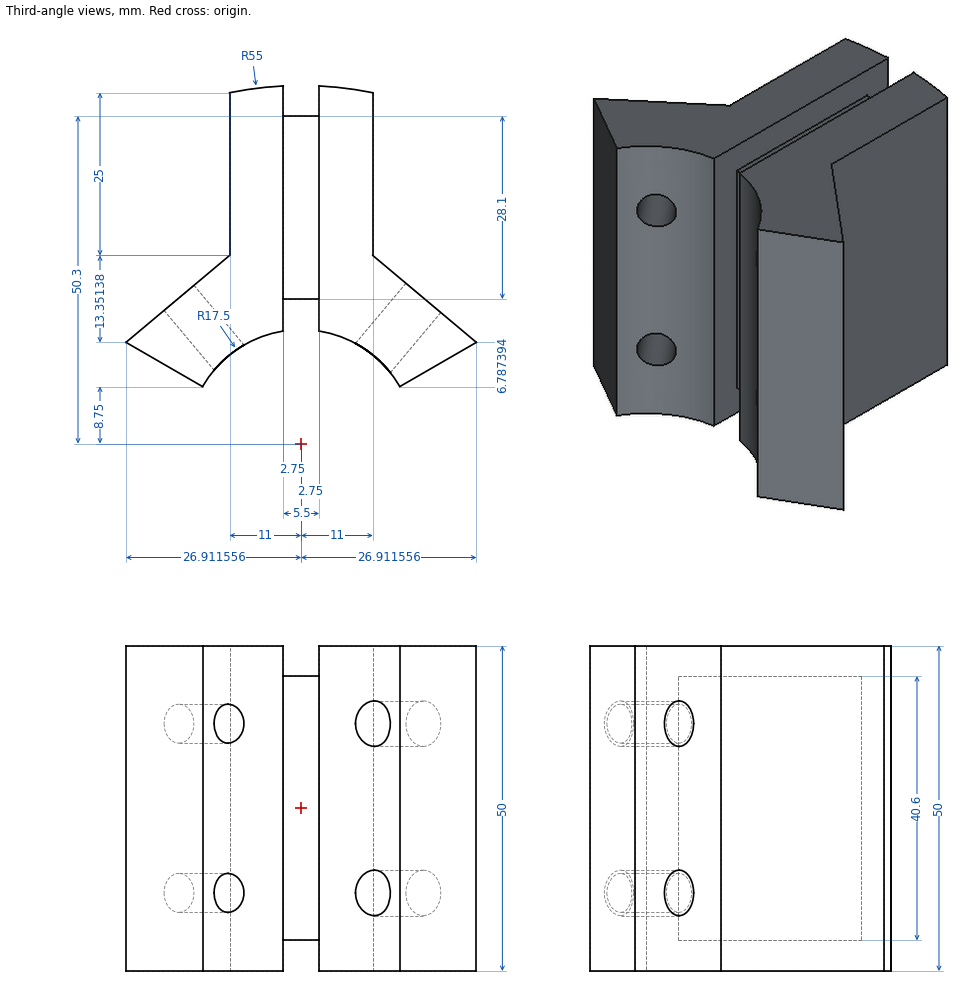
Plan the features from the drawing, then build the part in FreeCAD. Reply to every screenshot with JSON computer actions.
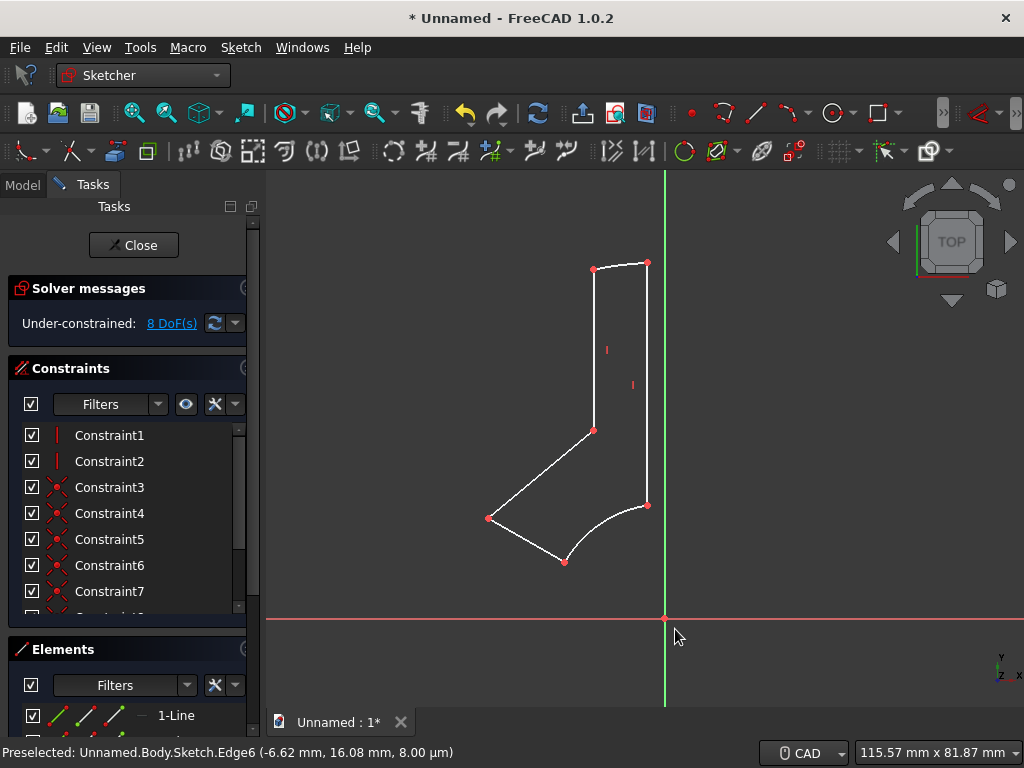
{"action": "left_click", "coordinate": [631, 264]}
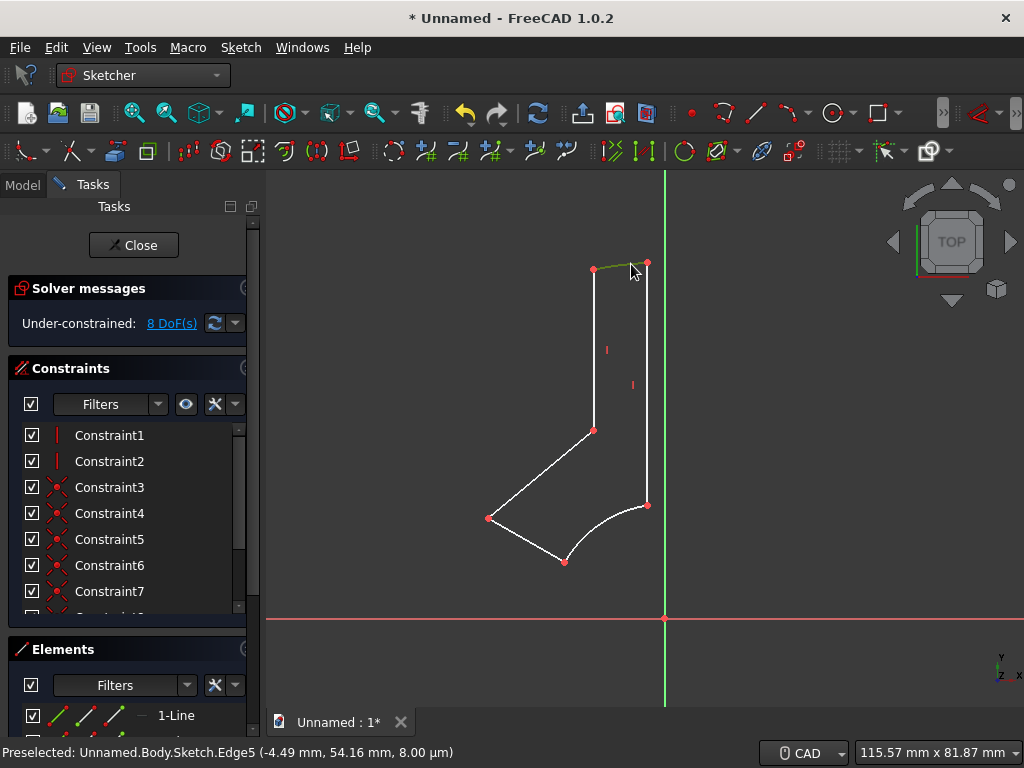
{"action": "left_click", "coordinate": [1002, 114]}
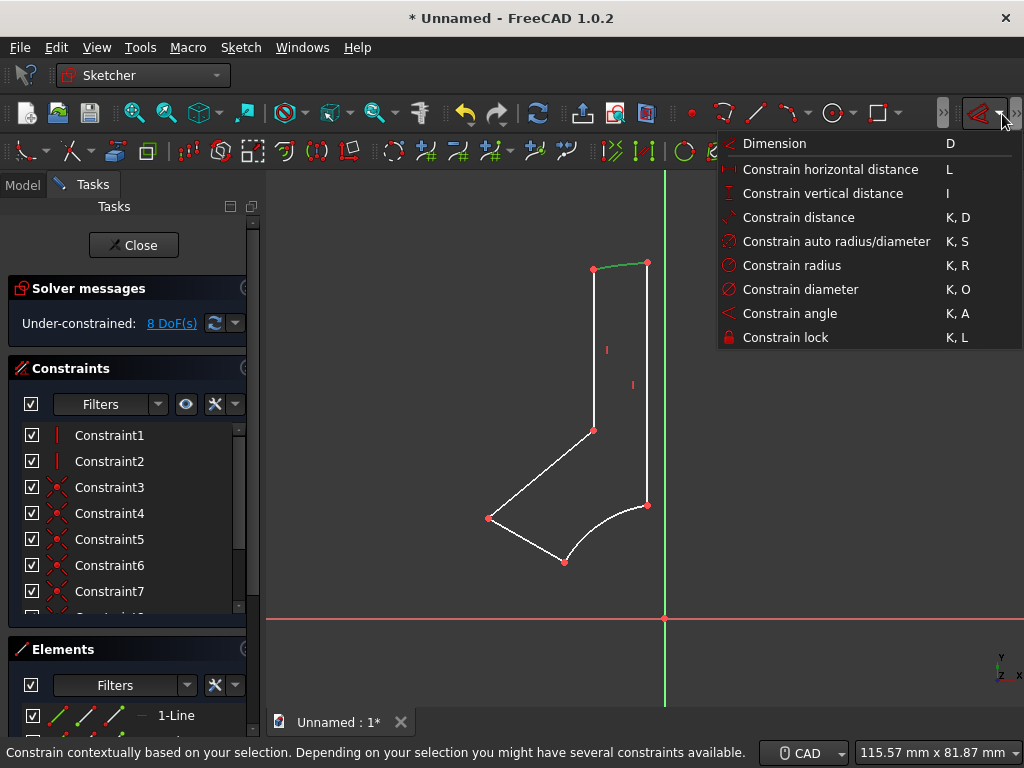
{"action": "left_click", "coordinate": [870, 265]}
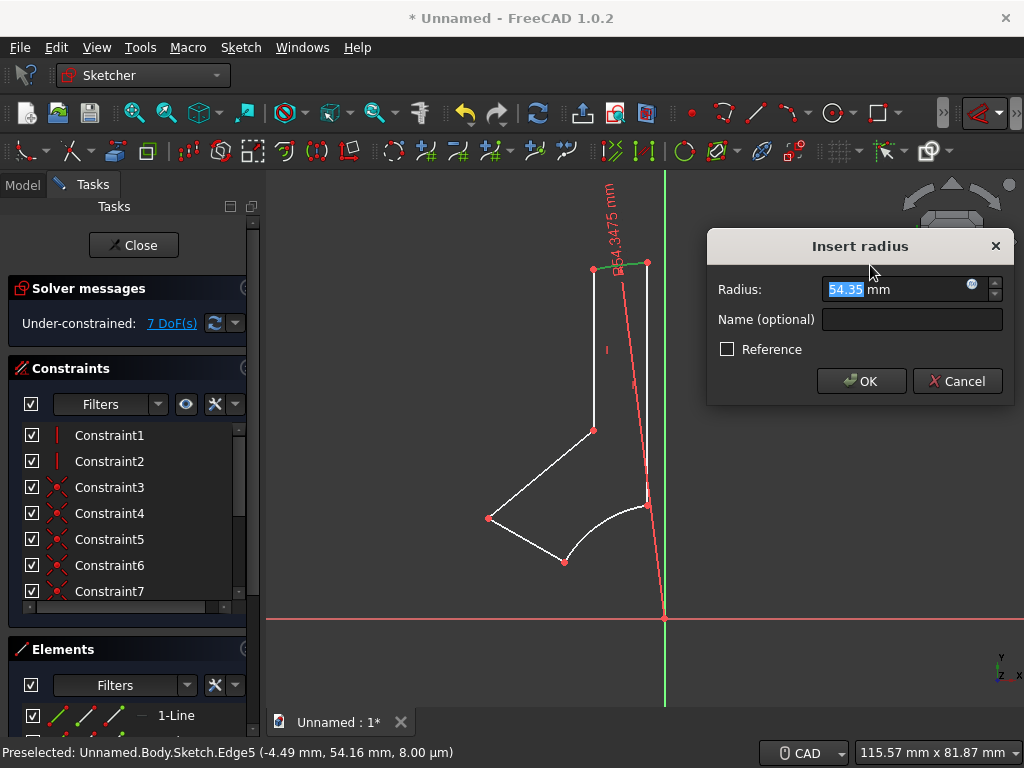
{"action": "type", "text": "55"}
{"action": "key", "text": "Return"}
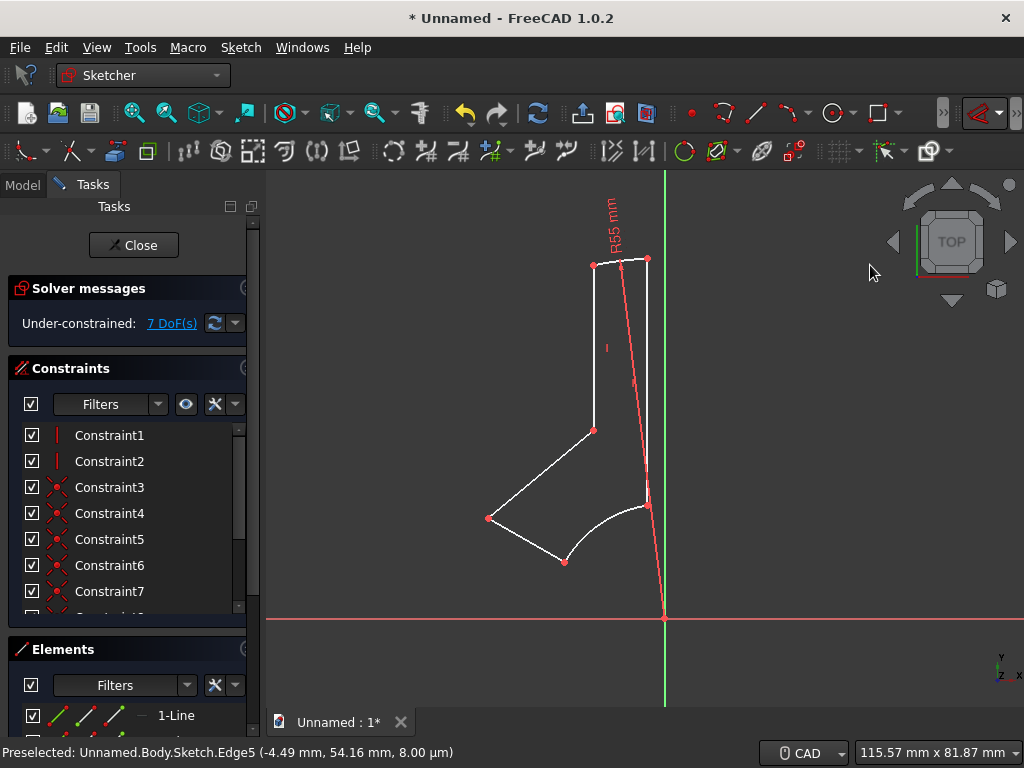
{"action": "left_click", "coordinate": [618, 514]}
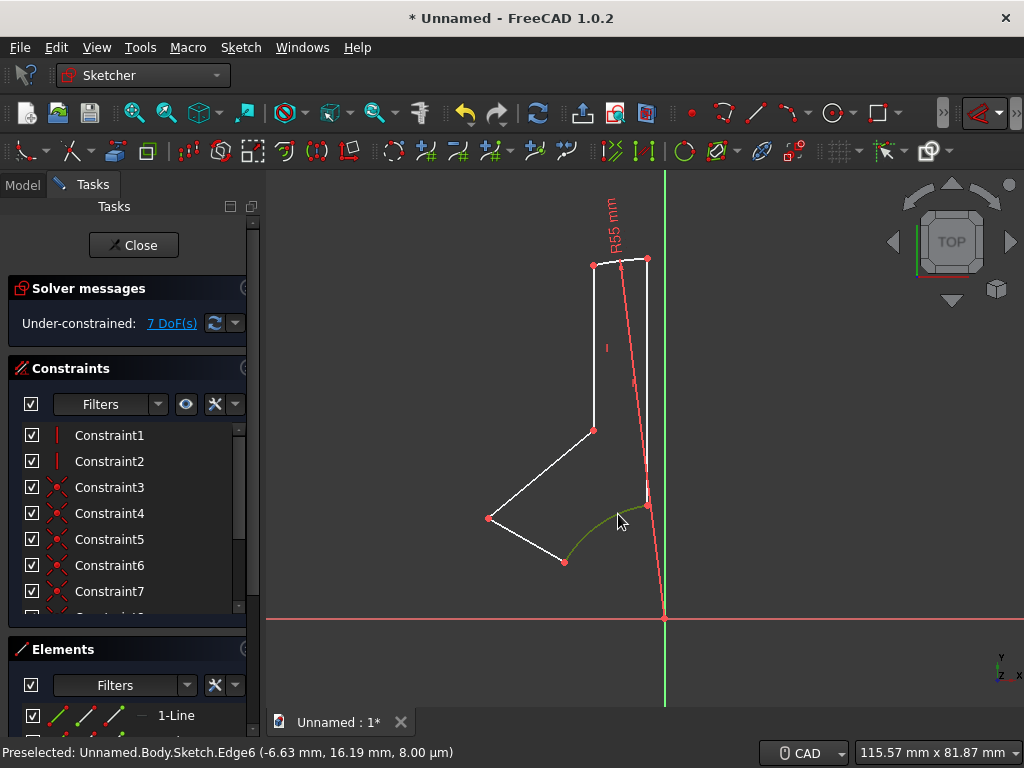
{"action": "key", "text": "k r"}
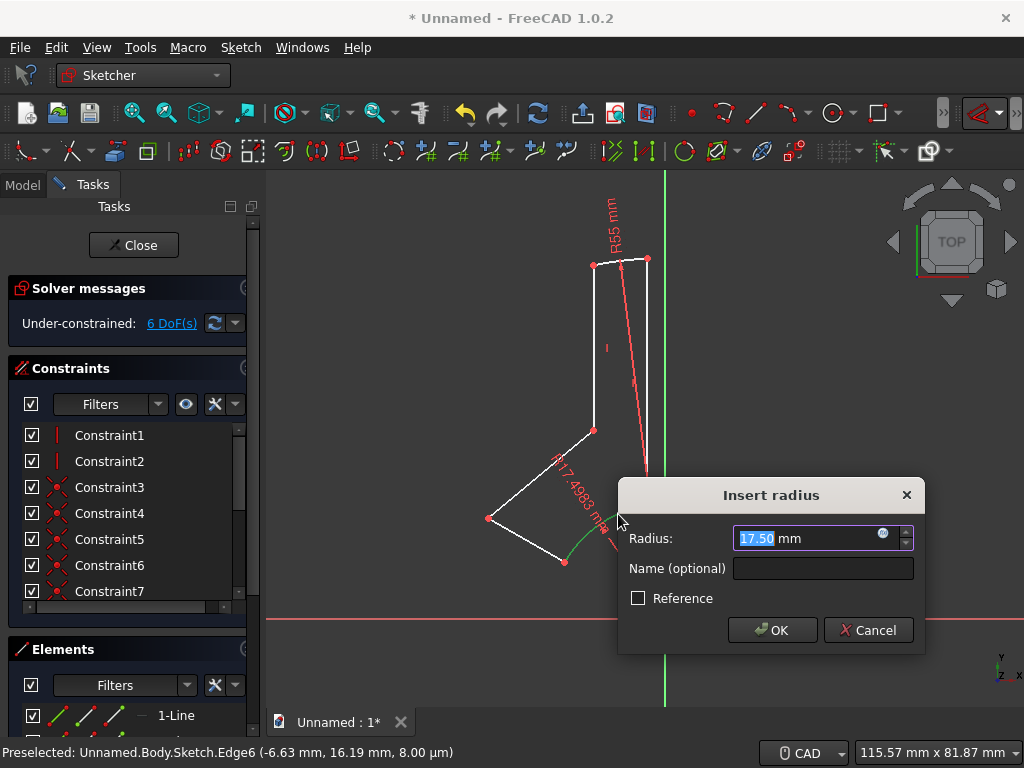
{"action": "type", "text": "17.5"}
{"action": "key", "text": "Return"}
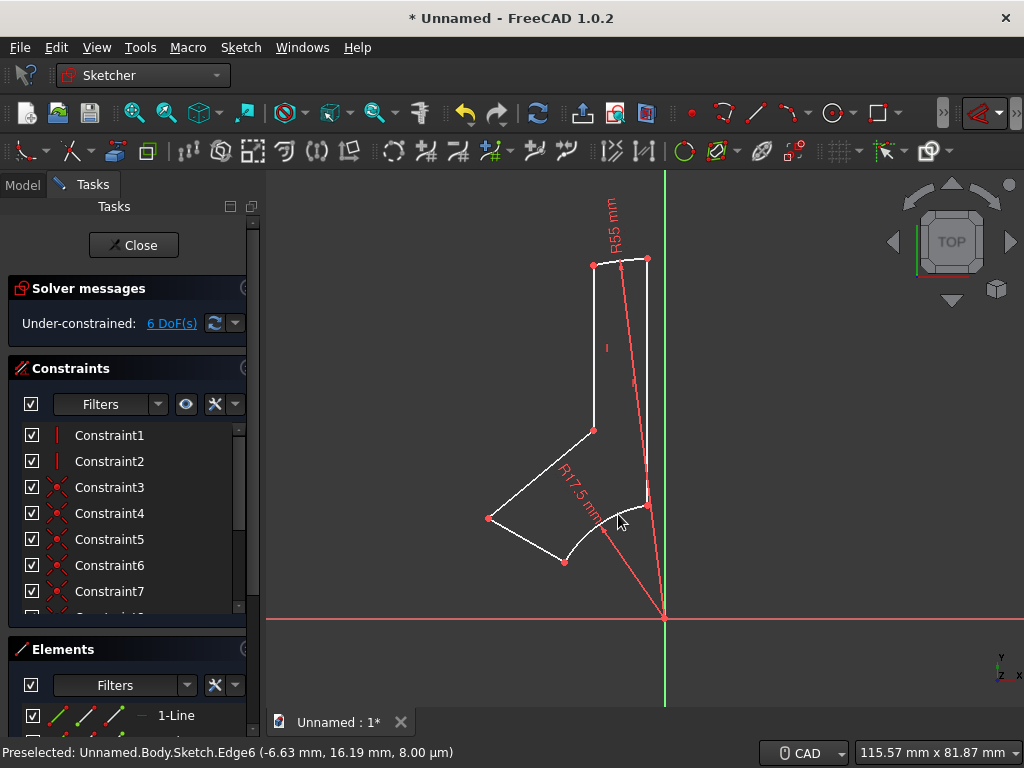
{"action": "left_click", "coordinate": [594, 315]}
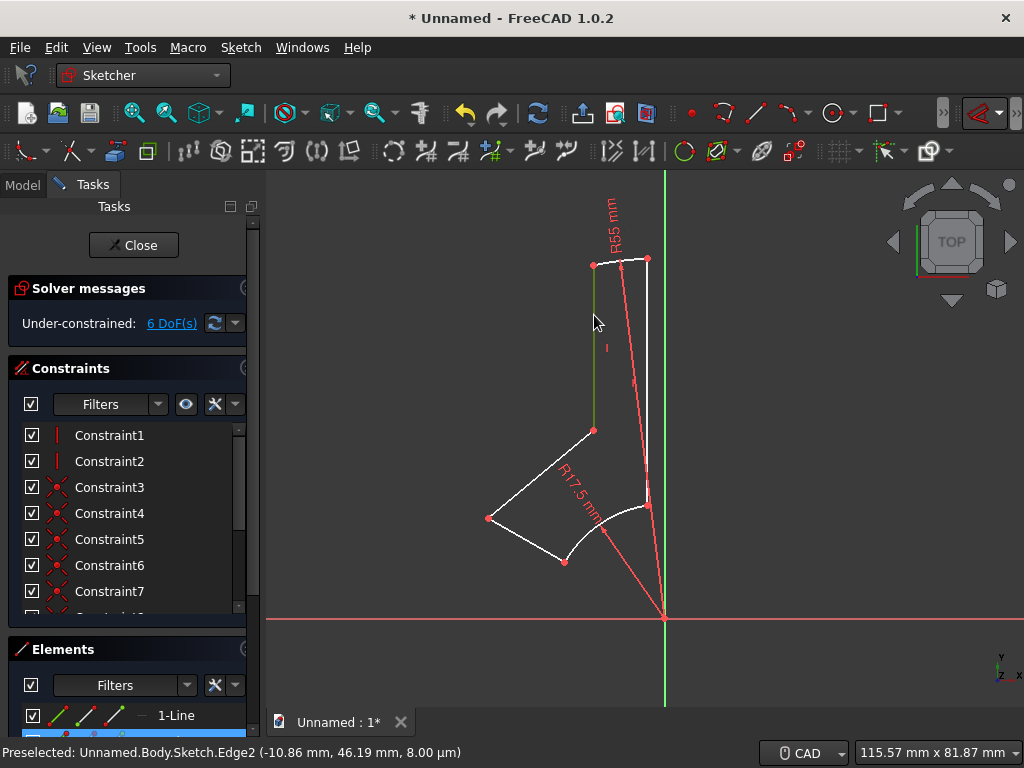
{"action": "left_click", "coordinate": [1002, 114]}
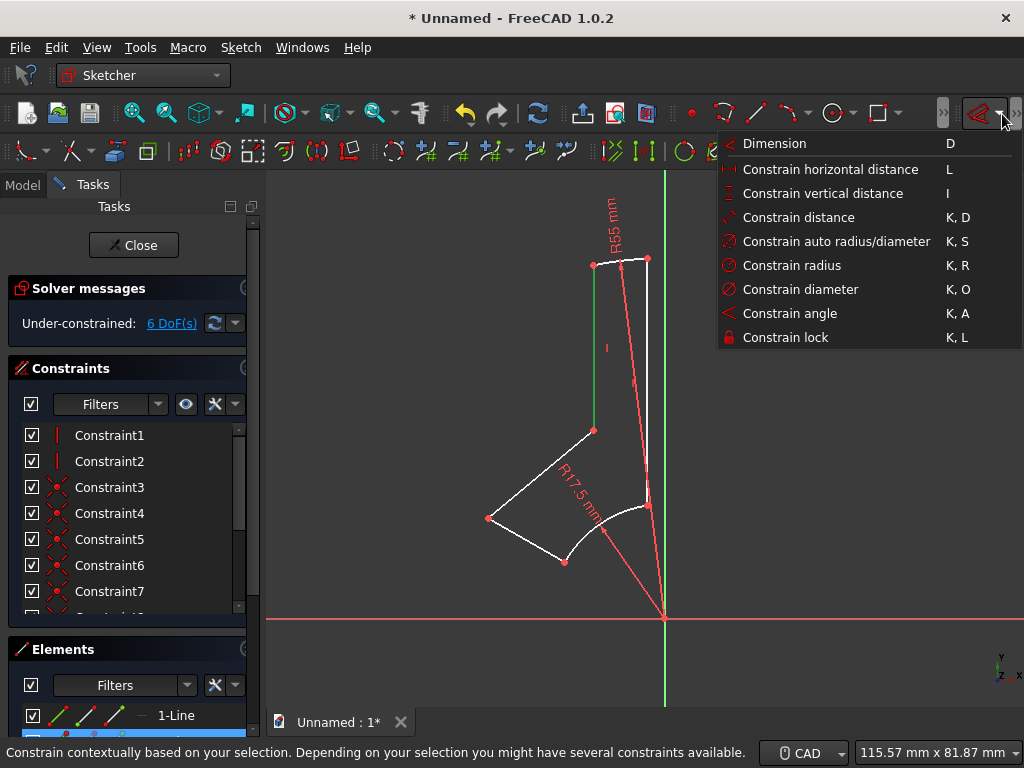
{"action": "left_click", "coordinate": [870, 193]}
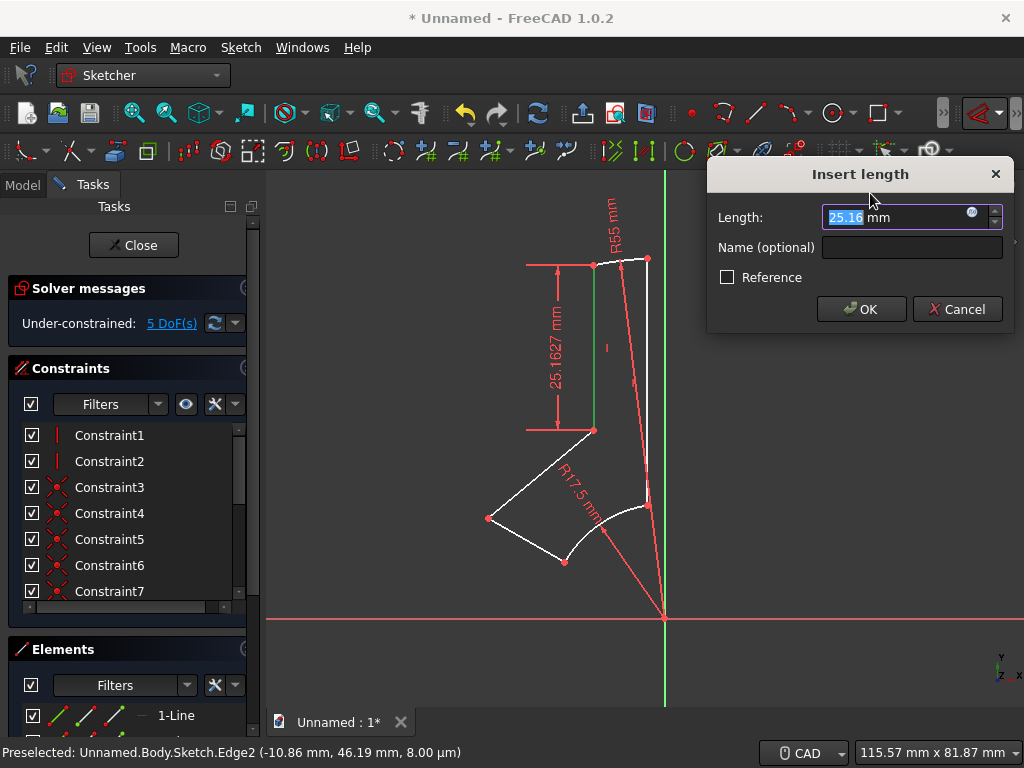
{"action": "type", "text": "25"}
{"action": "key", "text": "Return"}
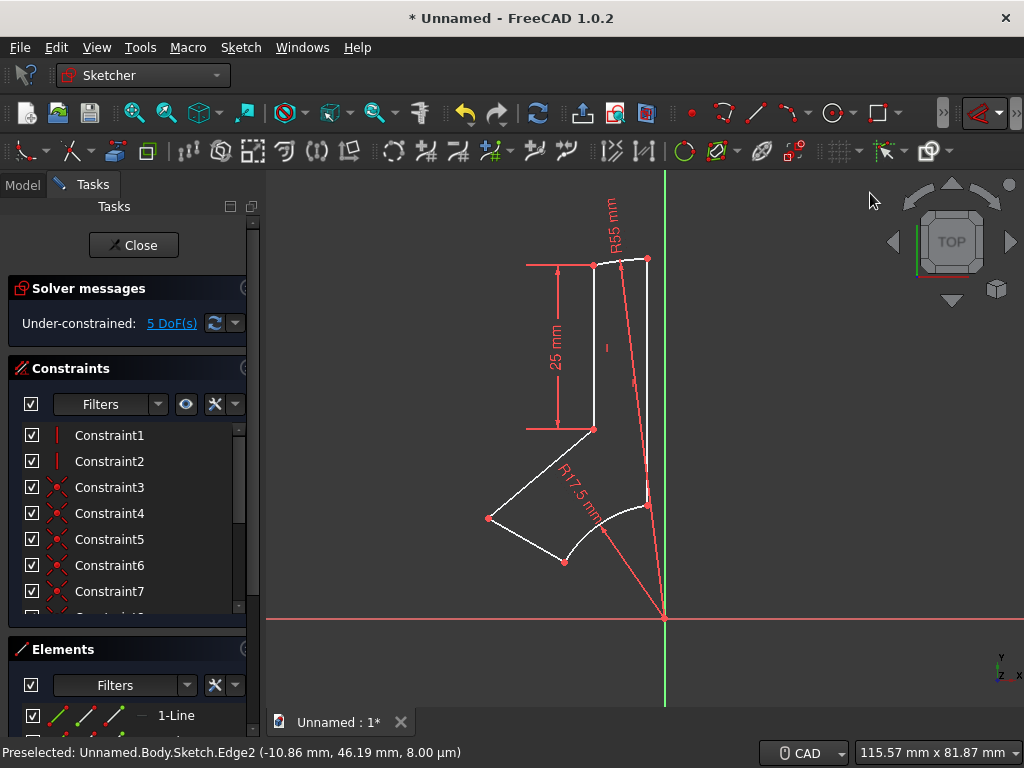
{"action": "left_click", "coordinate": [594, 265]}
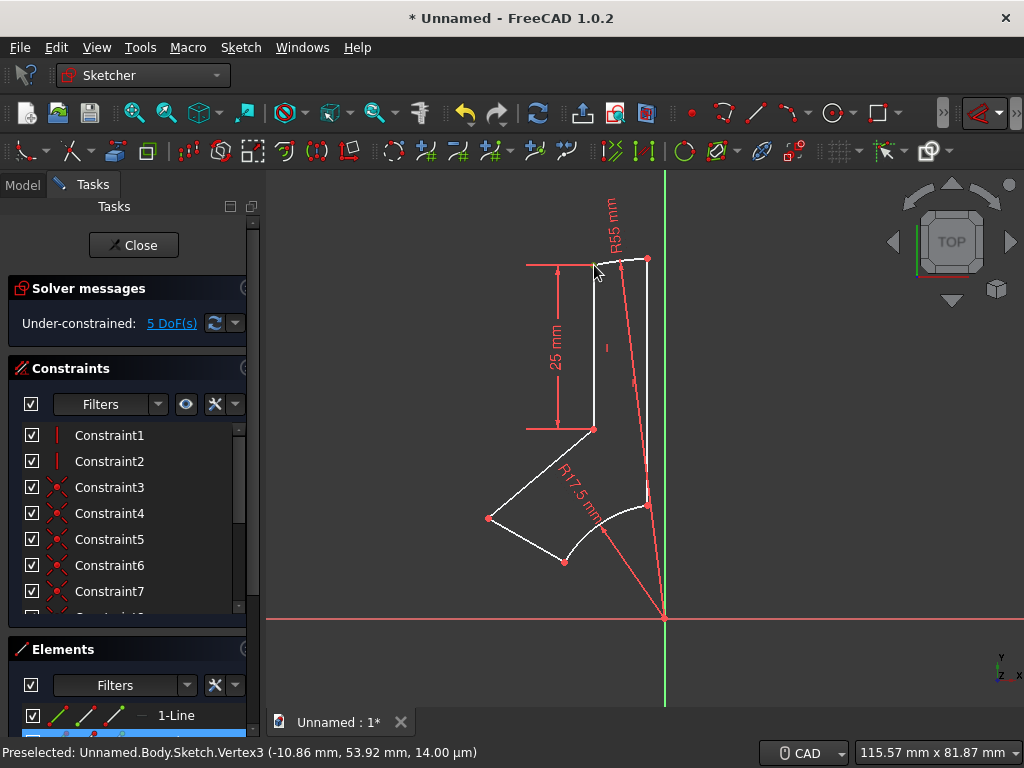
{"action": "left_click", "coordinate": [1002, 114]}